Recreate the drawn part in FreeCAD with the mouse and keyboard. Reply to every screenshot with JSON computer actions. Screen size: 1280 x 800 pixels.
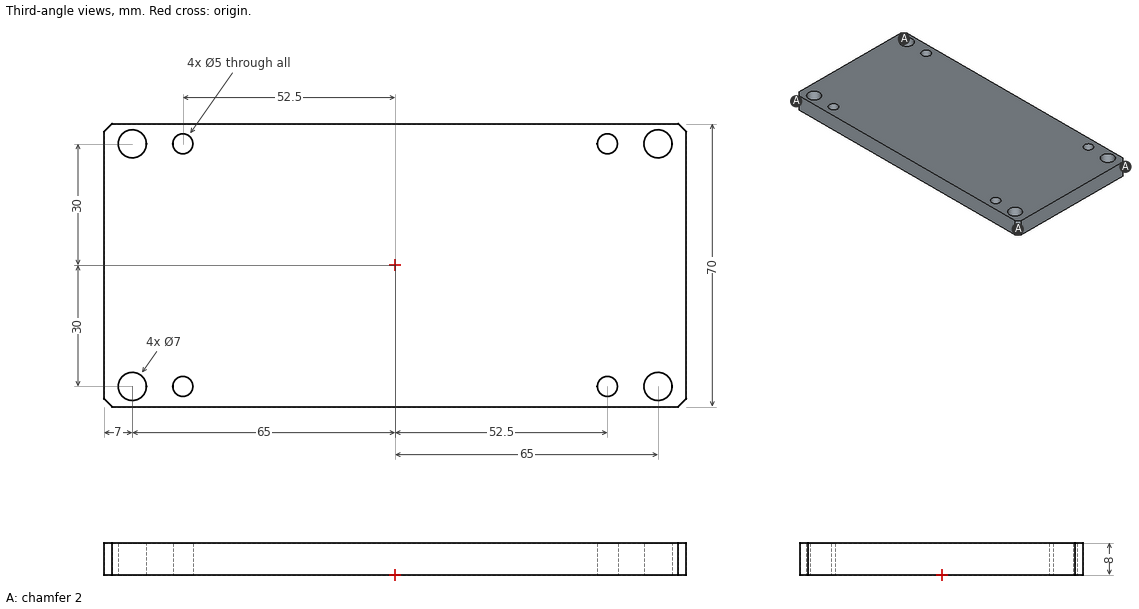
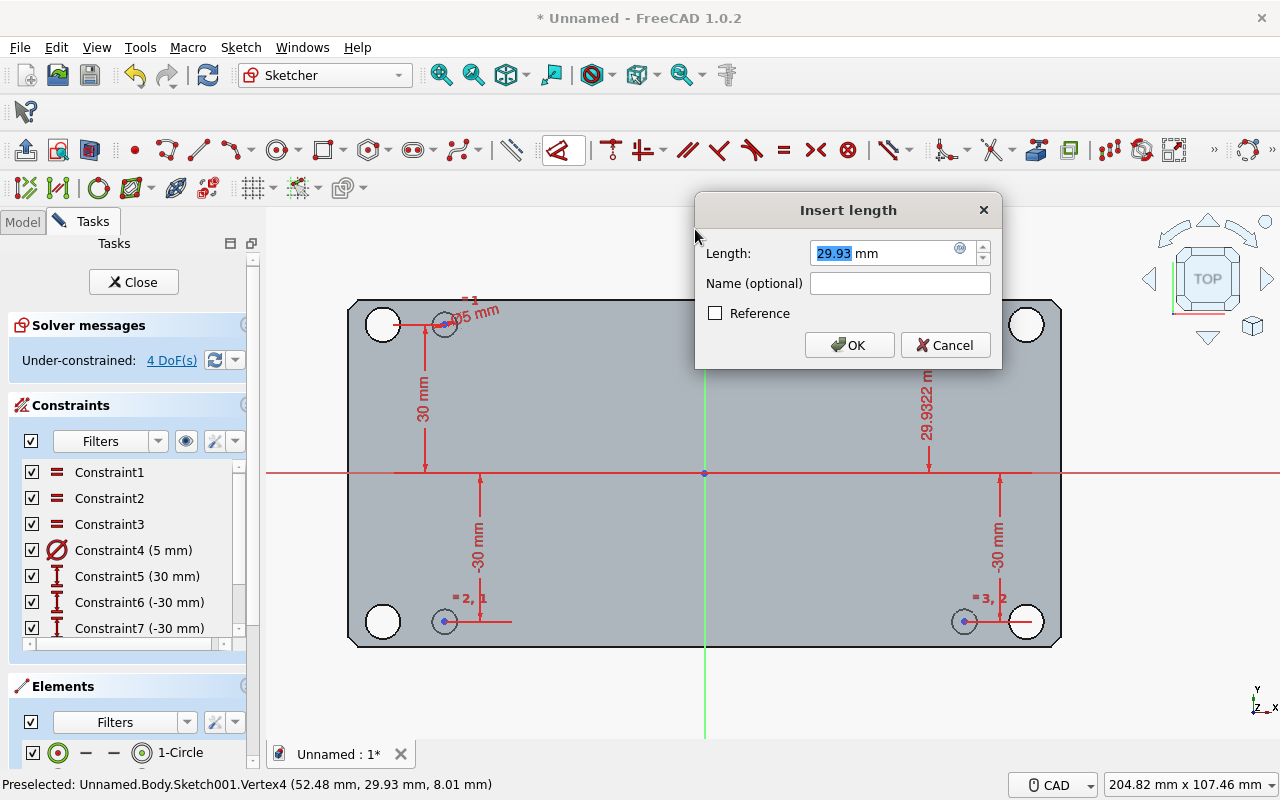
{"action": "type", "text": "30"}
{"action": "key", "text": "Return"}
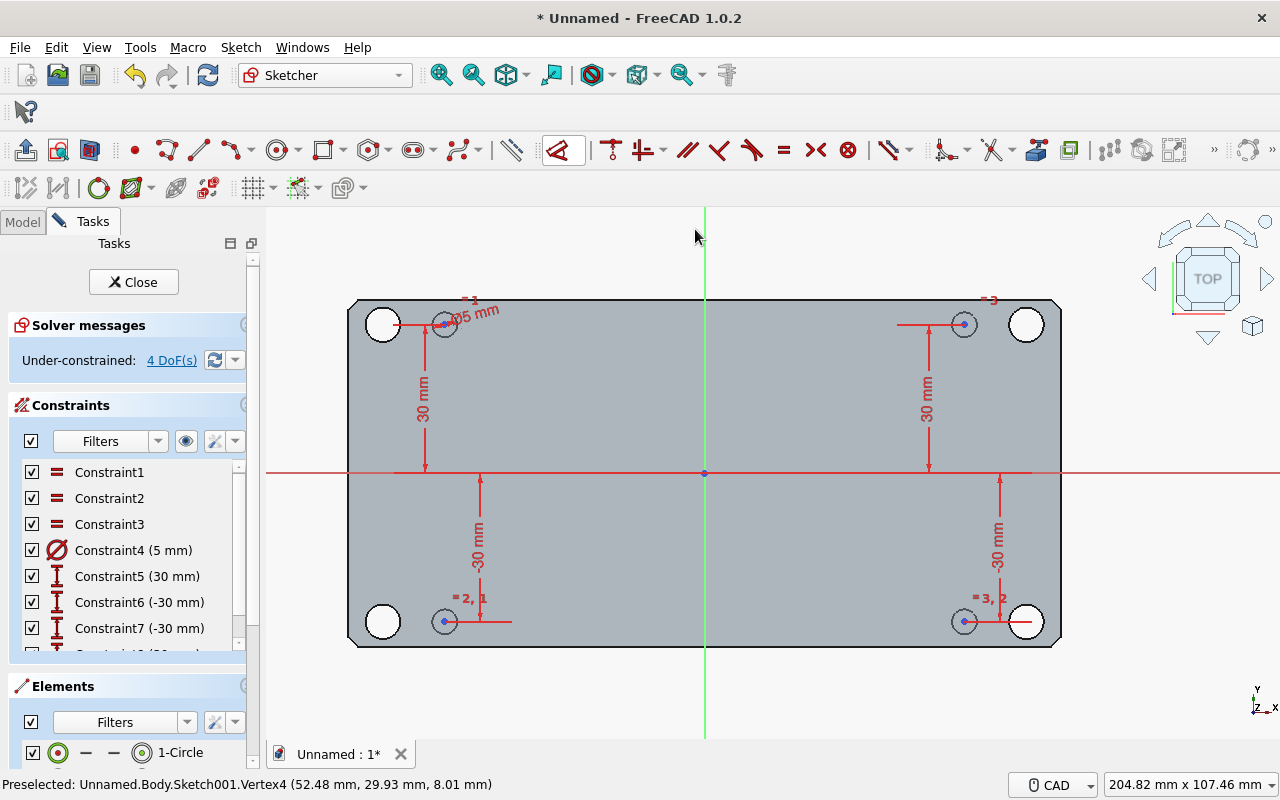
{"action": "left_click", "coordinate": [445, 325]}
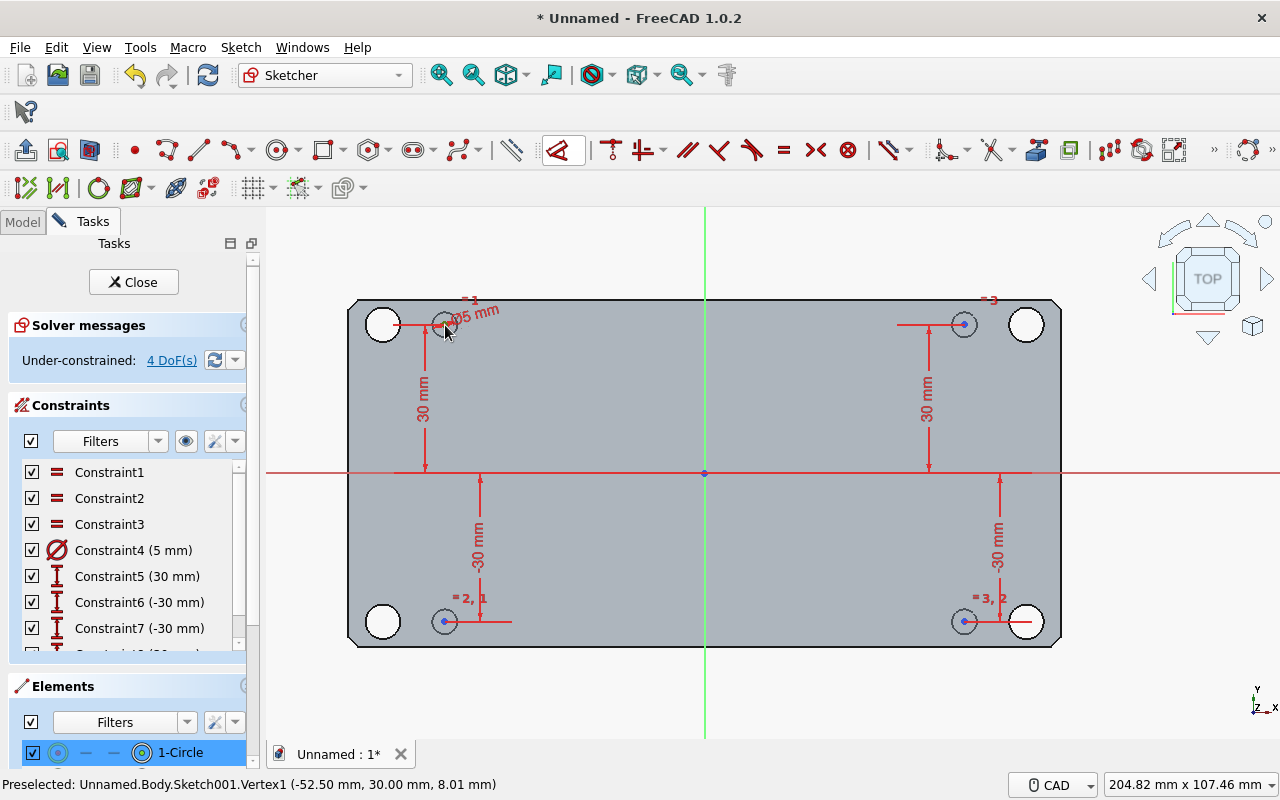
{"action": "left_click", "coordinate": [580, 150]}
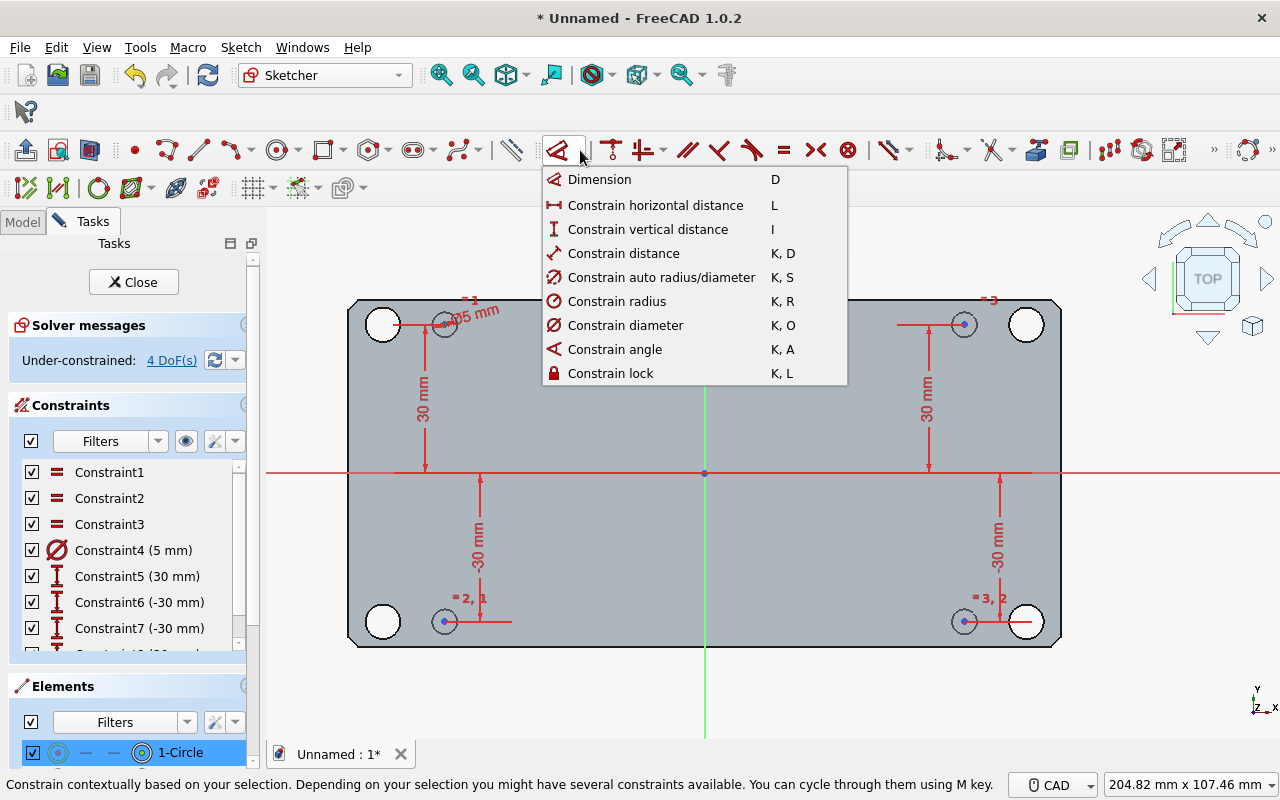
{"action": "left_click", "coordinate": [695, 205]}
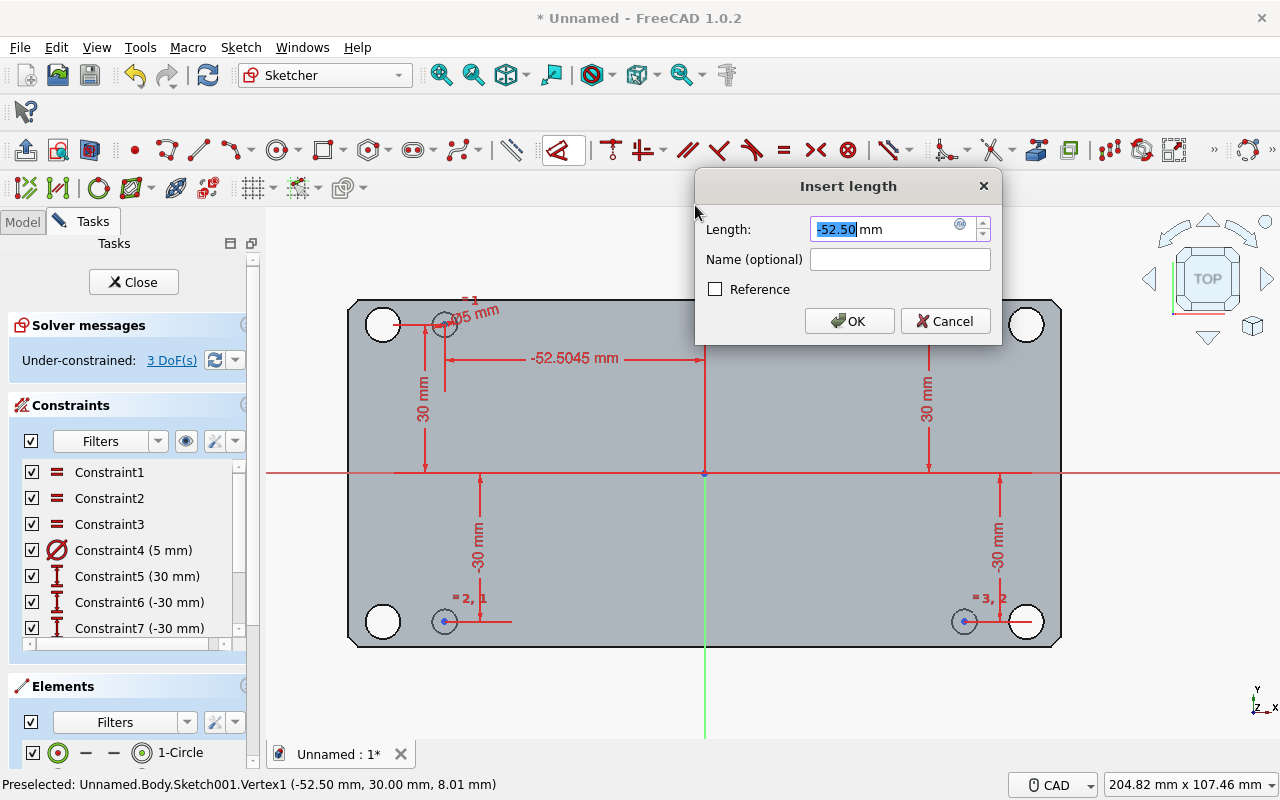
{"action": "type", "text": "-52.5"}
{"action": "key", "text": "Return"}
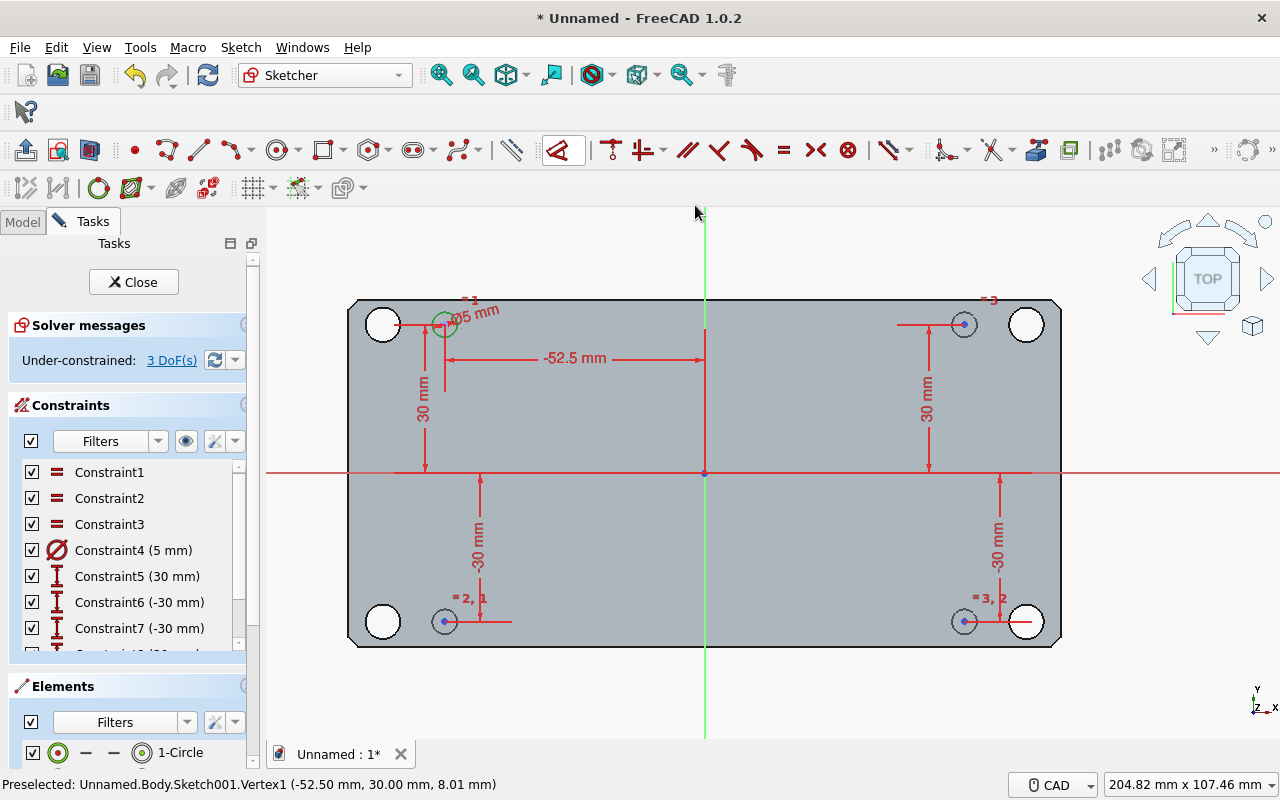
{"action": "left_click", "coordinate": [445, 622]}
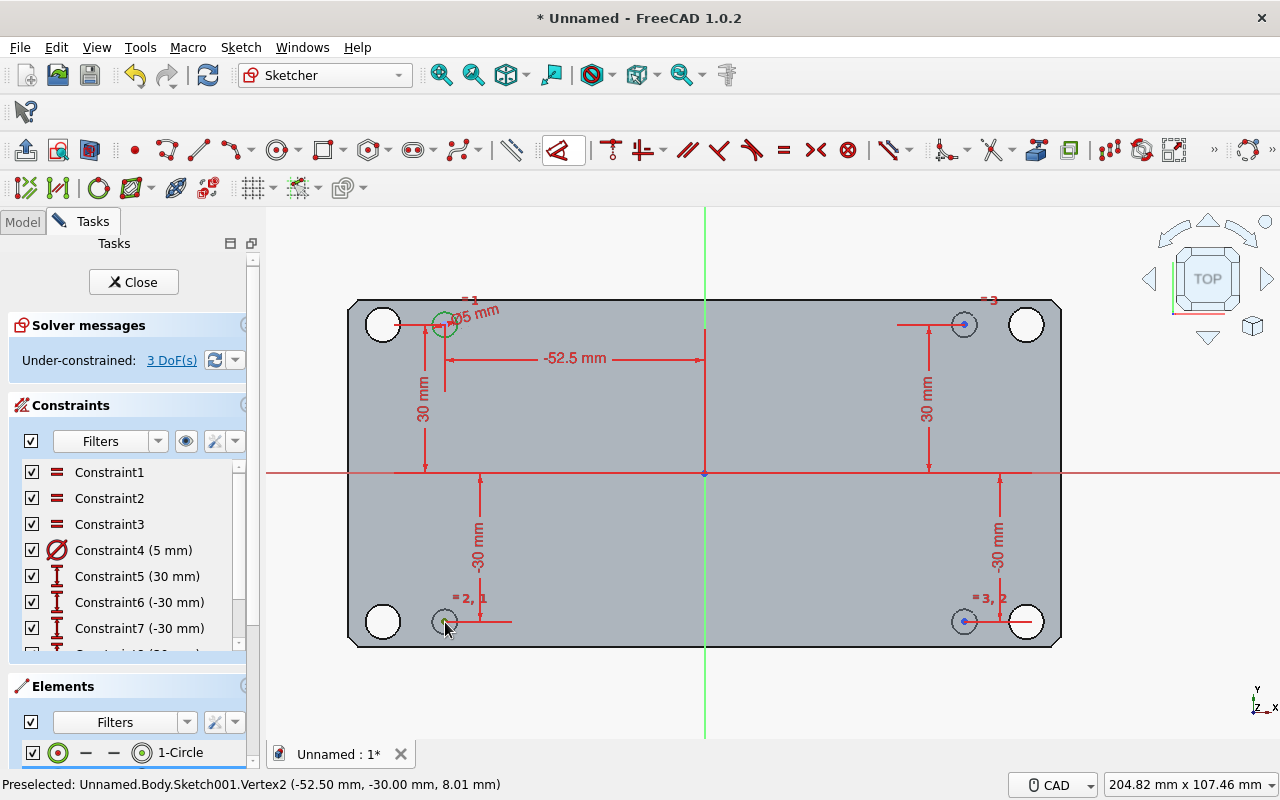
{"action": "left_click", "coordinate": [580, 150]}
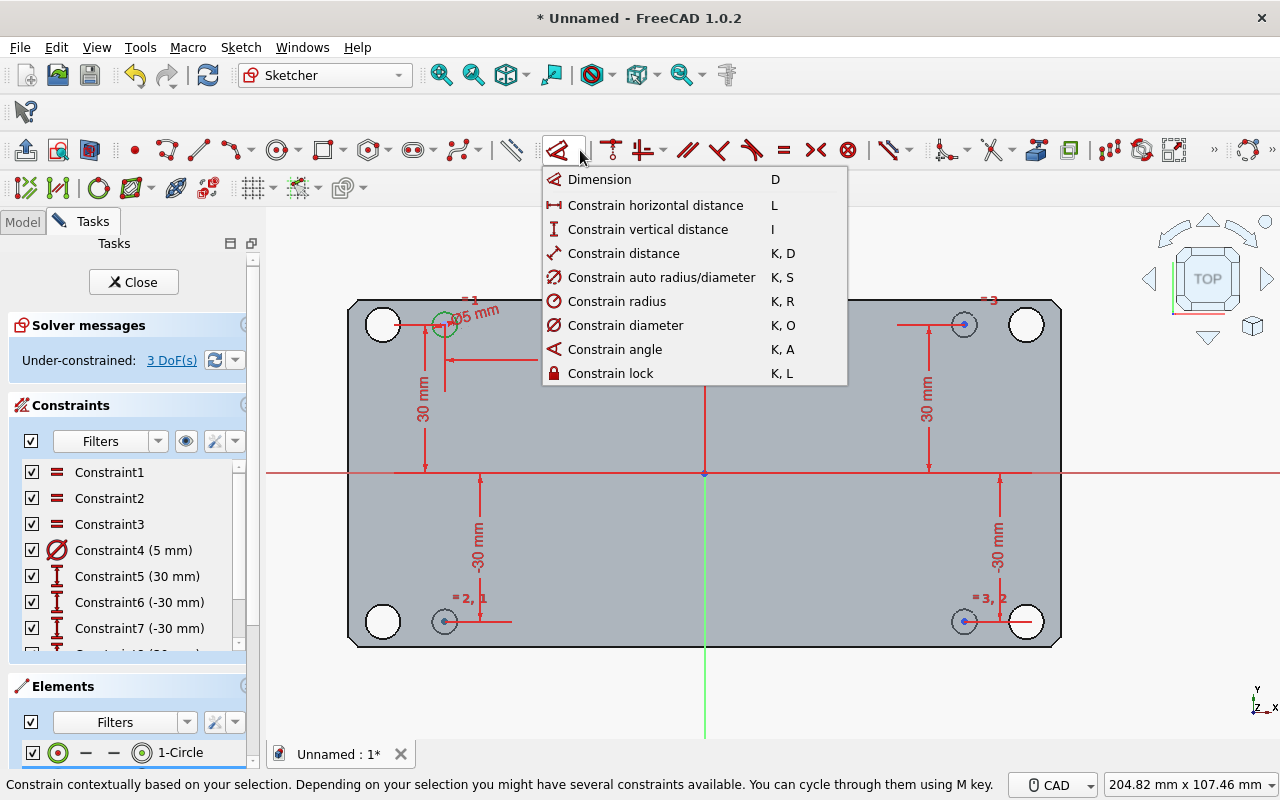
{"action": "left_click", "coordinate": [695, 205]}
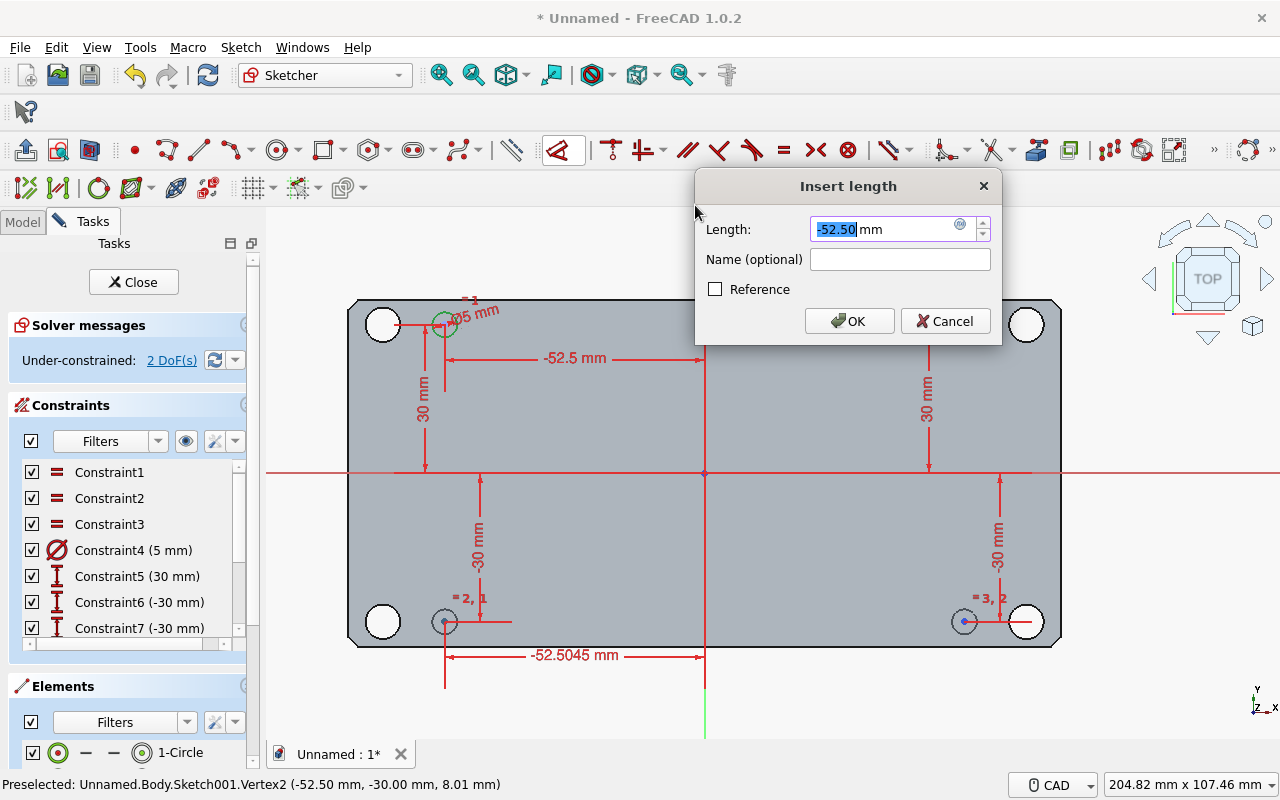
{"action": "type", "text": "-52.5"}
{"action": "key", "text": "Return"}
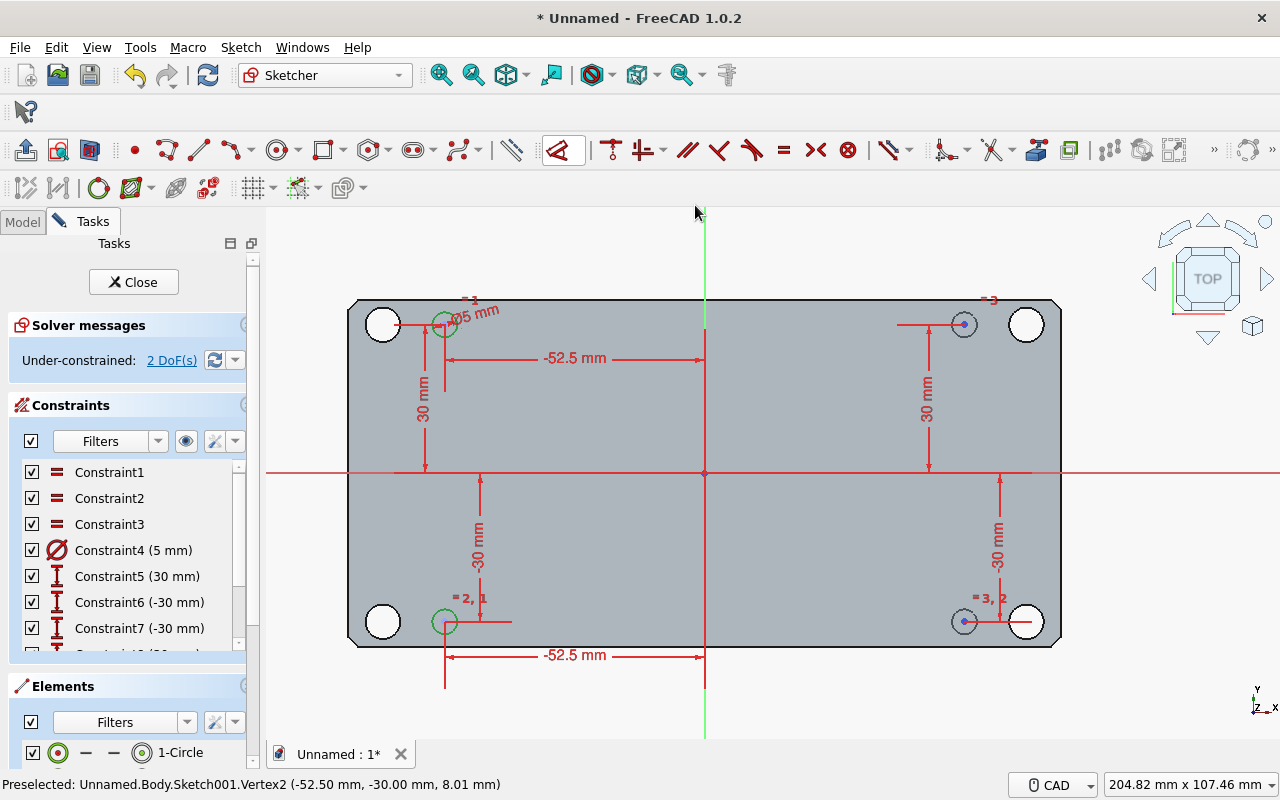
{"action": "left_click", "coordinate": [964, 622]}